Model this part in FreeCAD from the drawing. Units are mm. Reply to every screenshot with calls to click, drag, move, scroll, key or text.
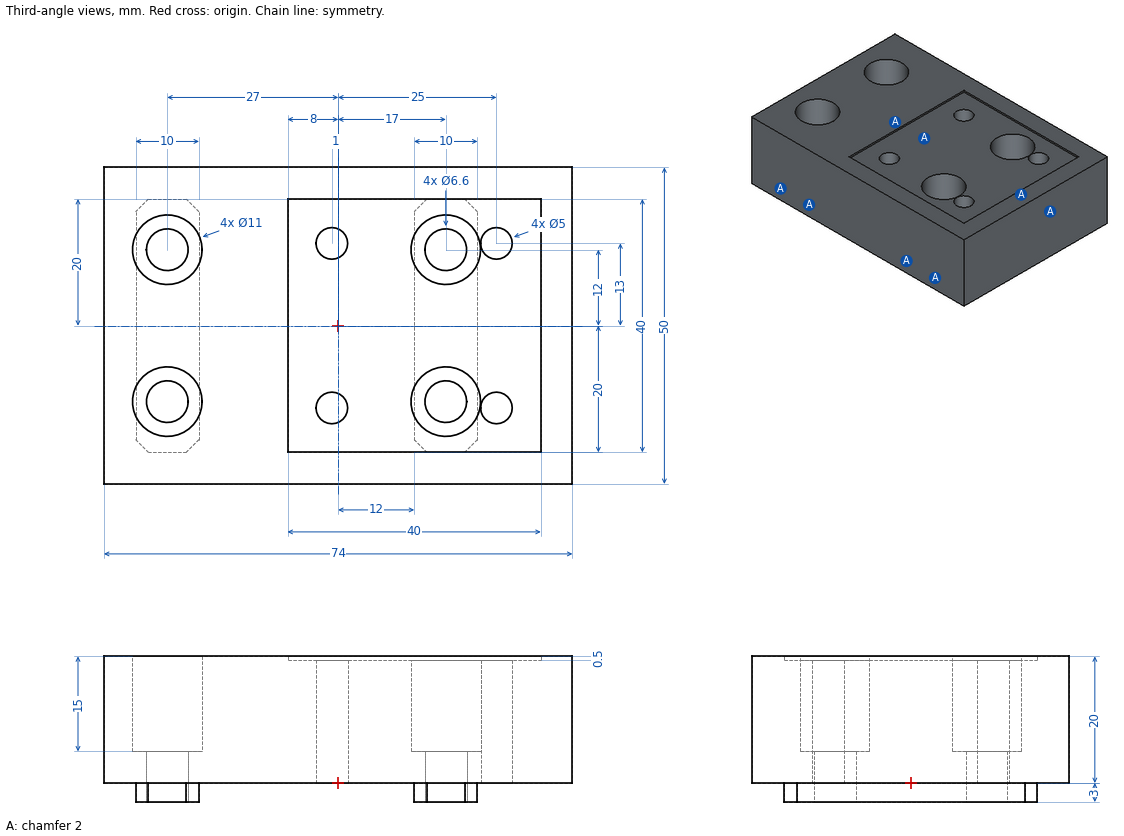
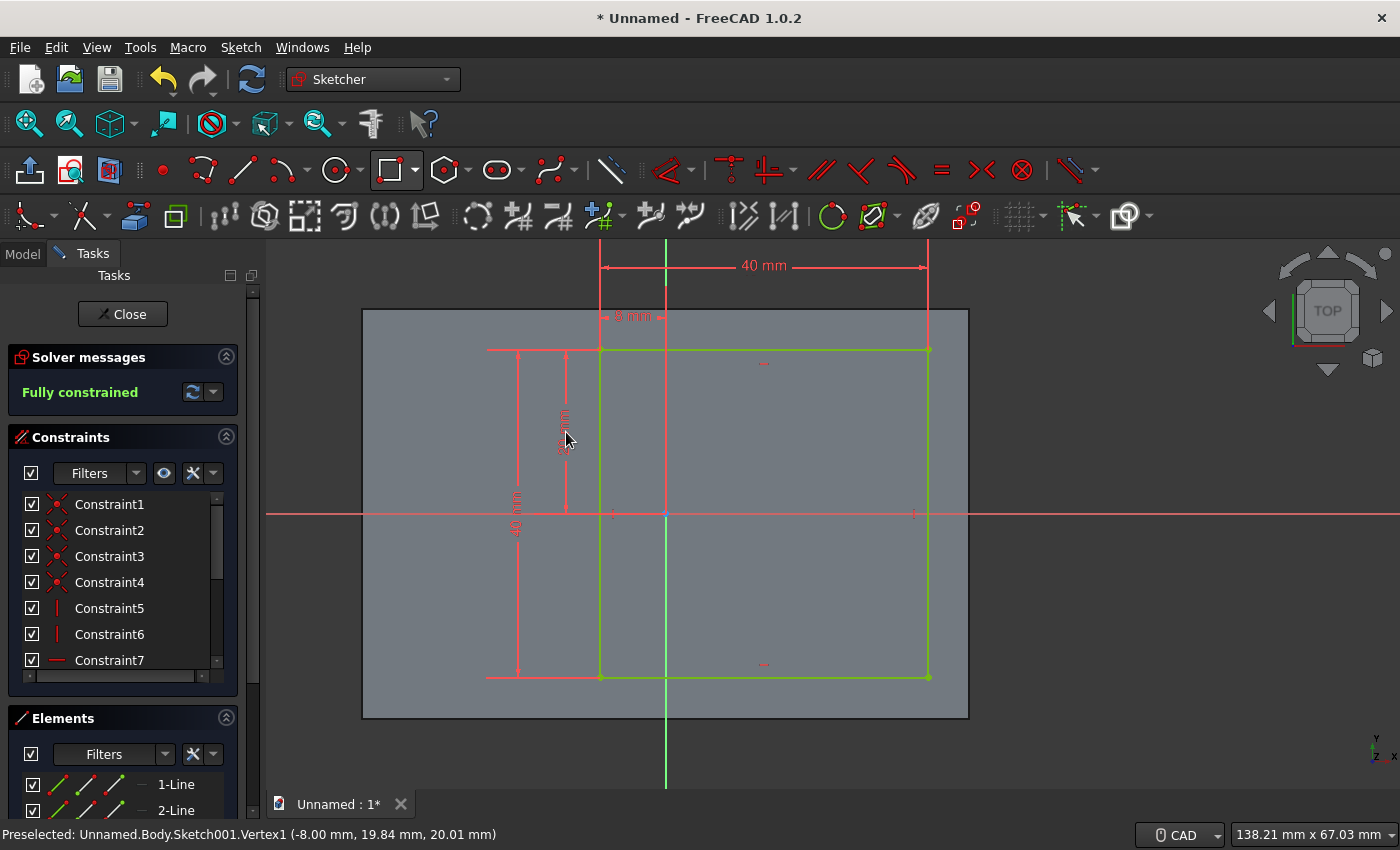
click(123, 314)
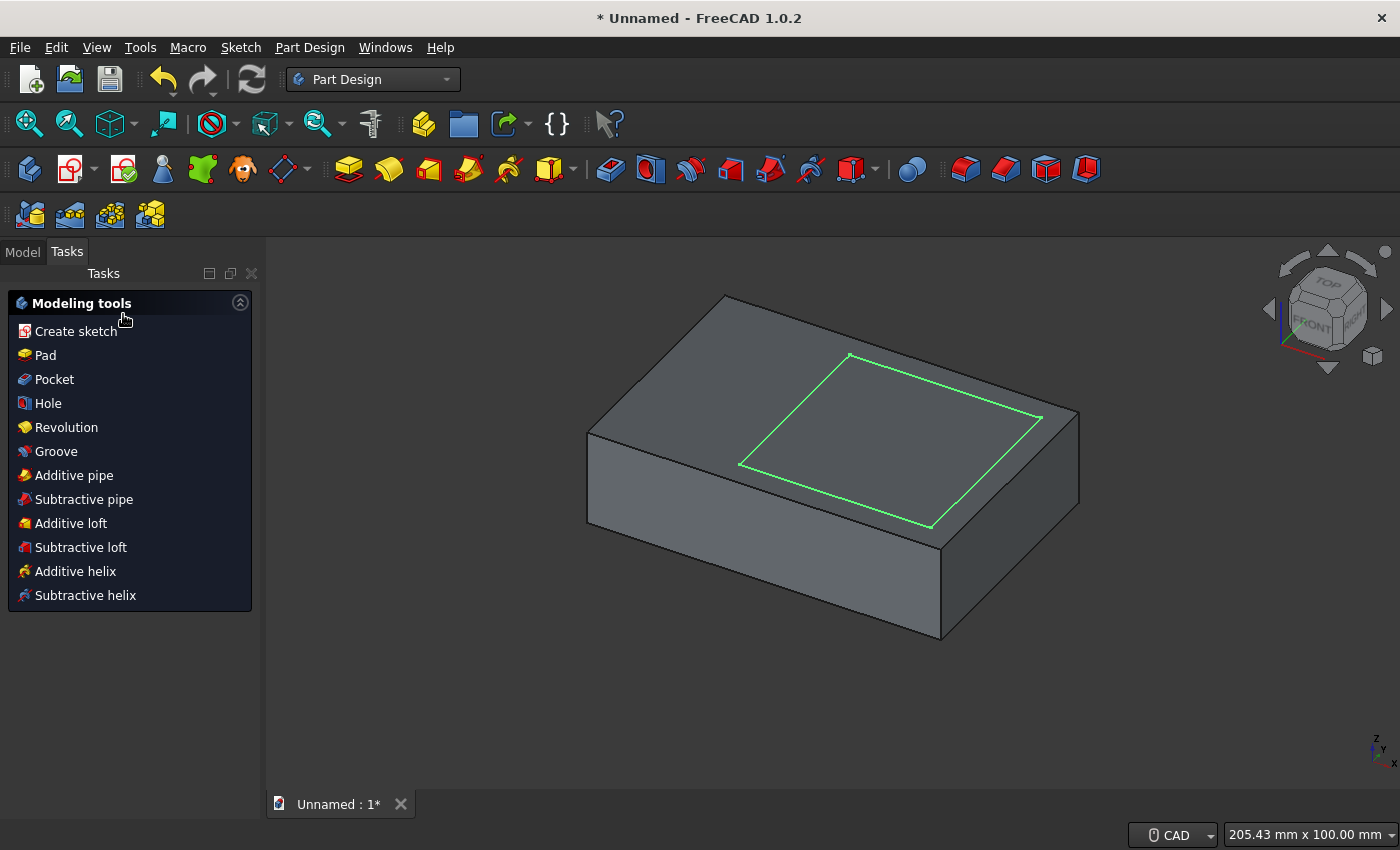
click(612, 170)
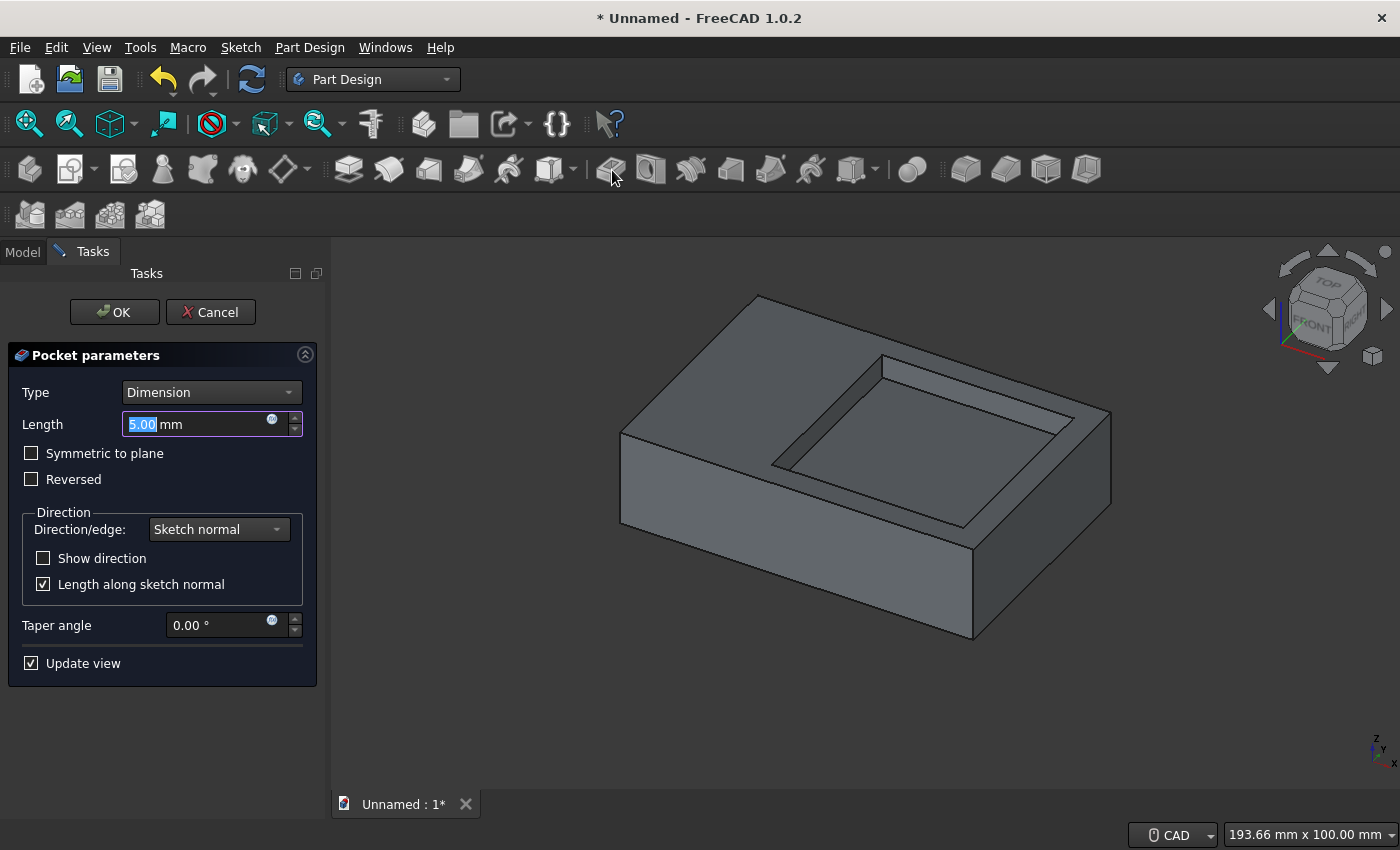
text(0.5)
key(Tab)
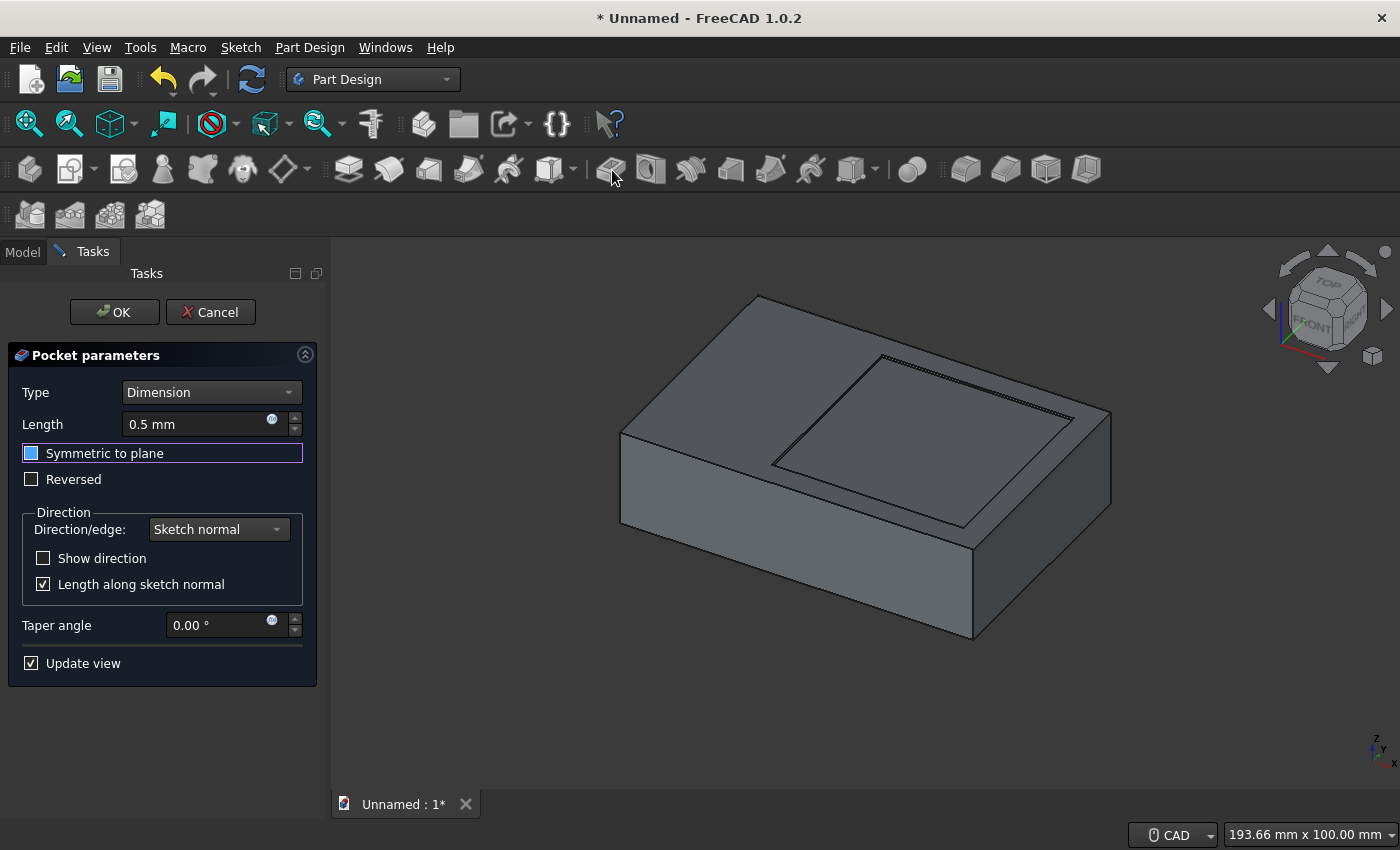
click(115, 312)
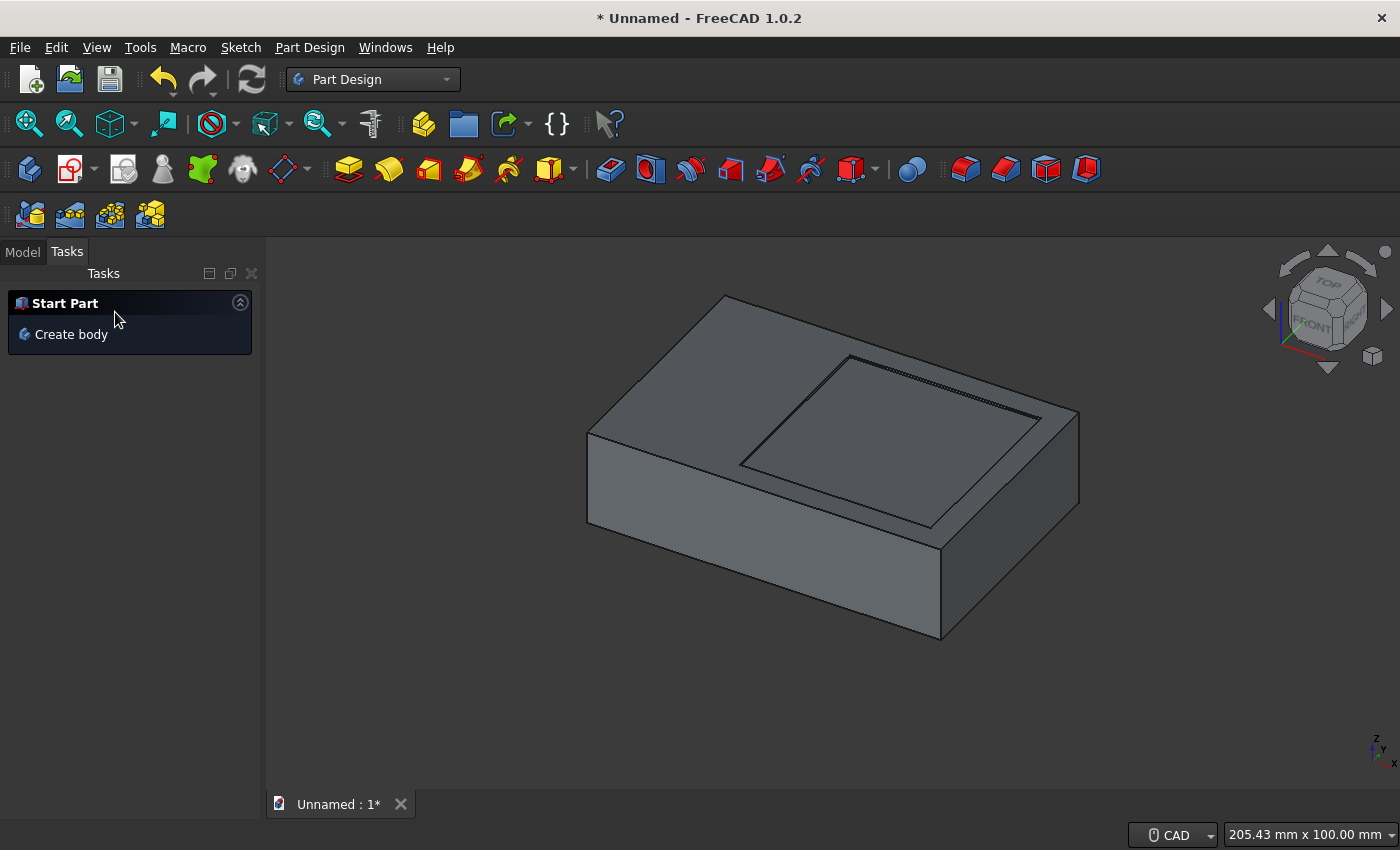
key(5)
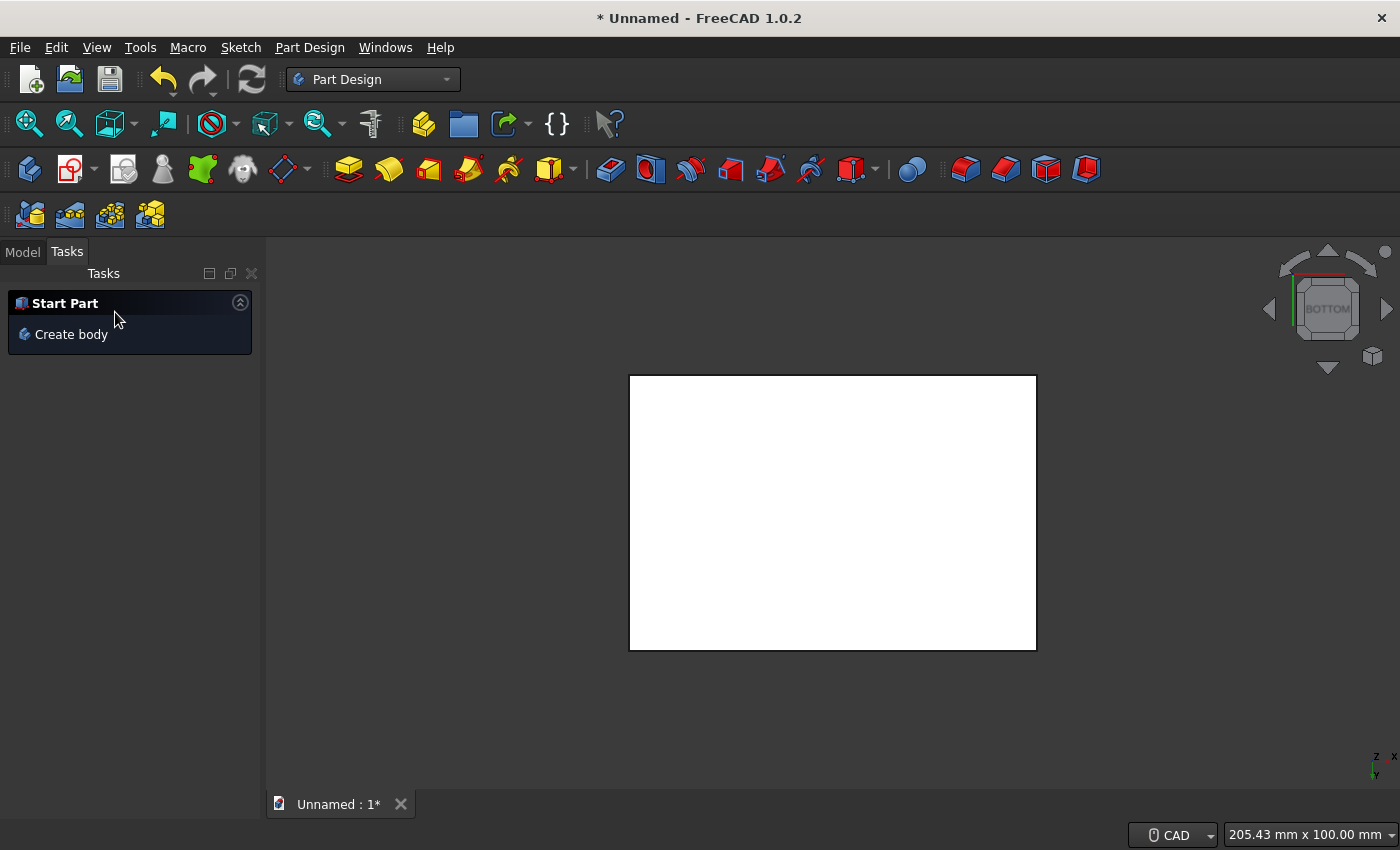
click(891, 512)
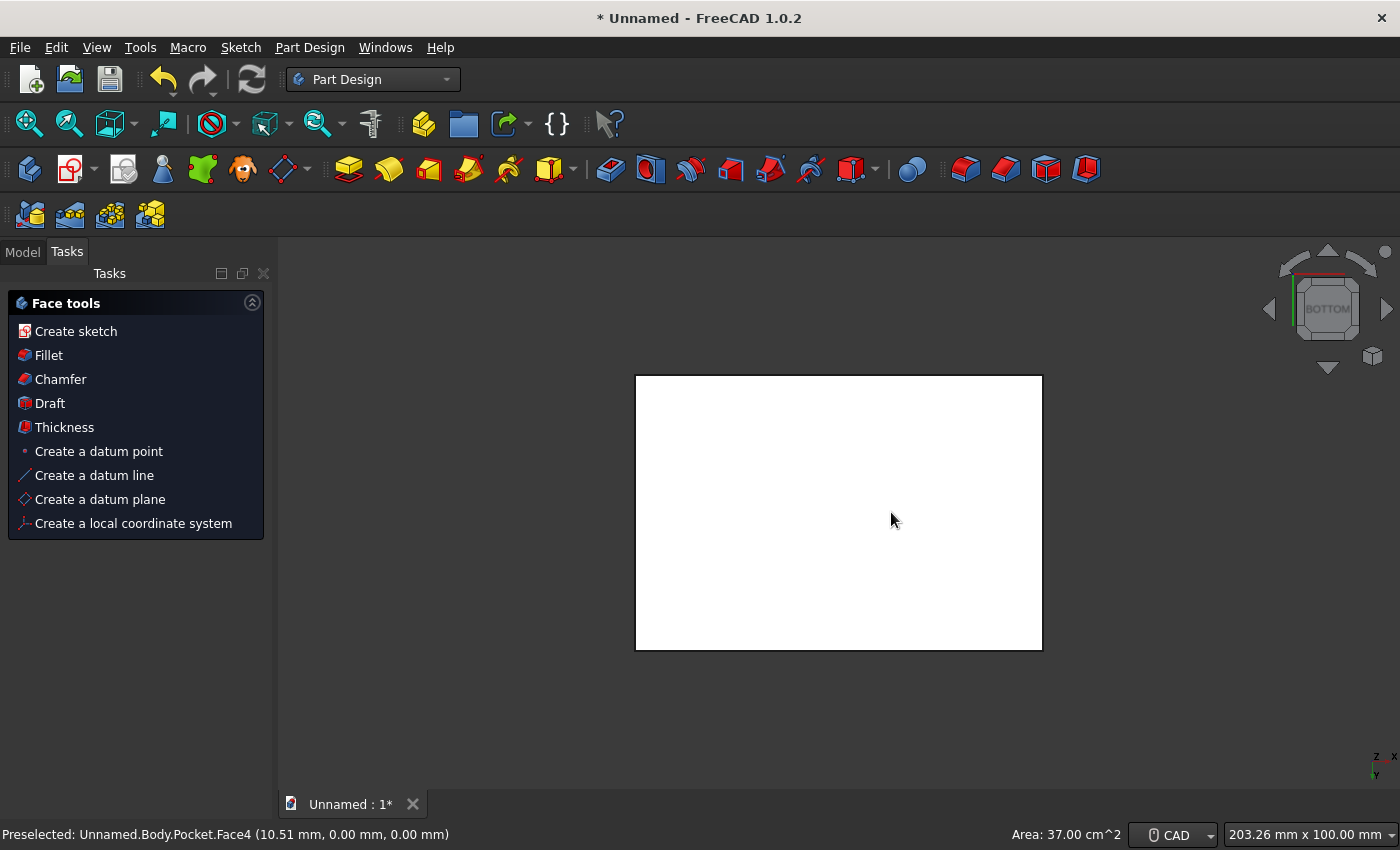
click(70, 170)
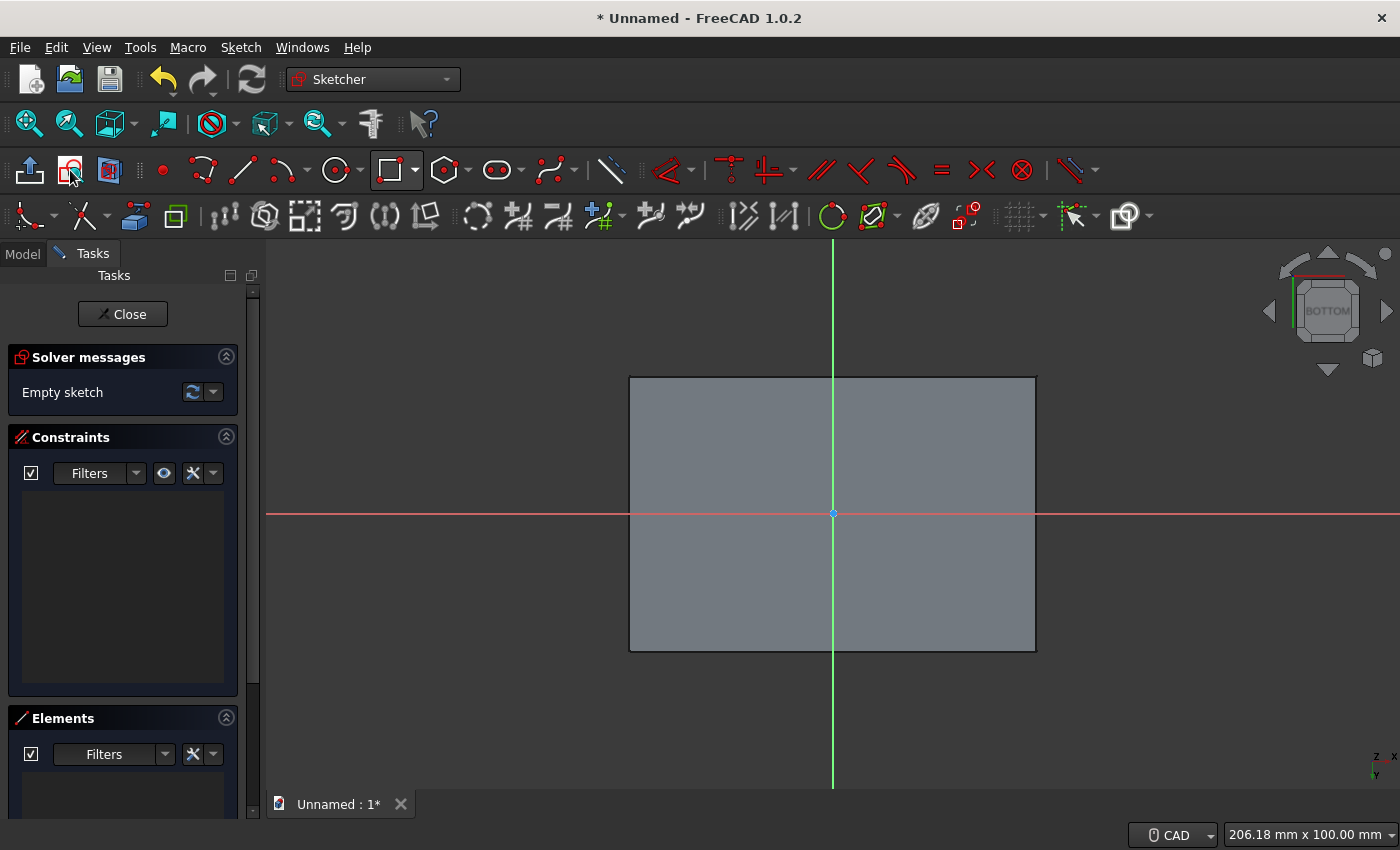
scroll(889, 514, up, 2)